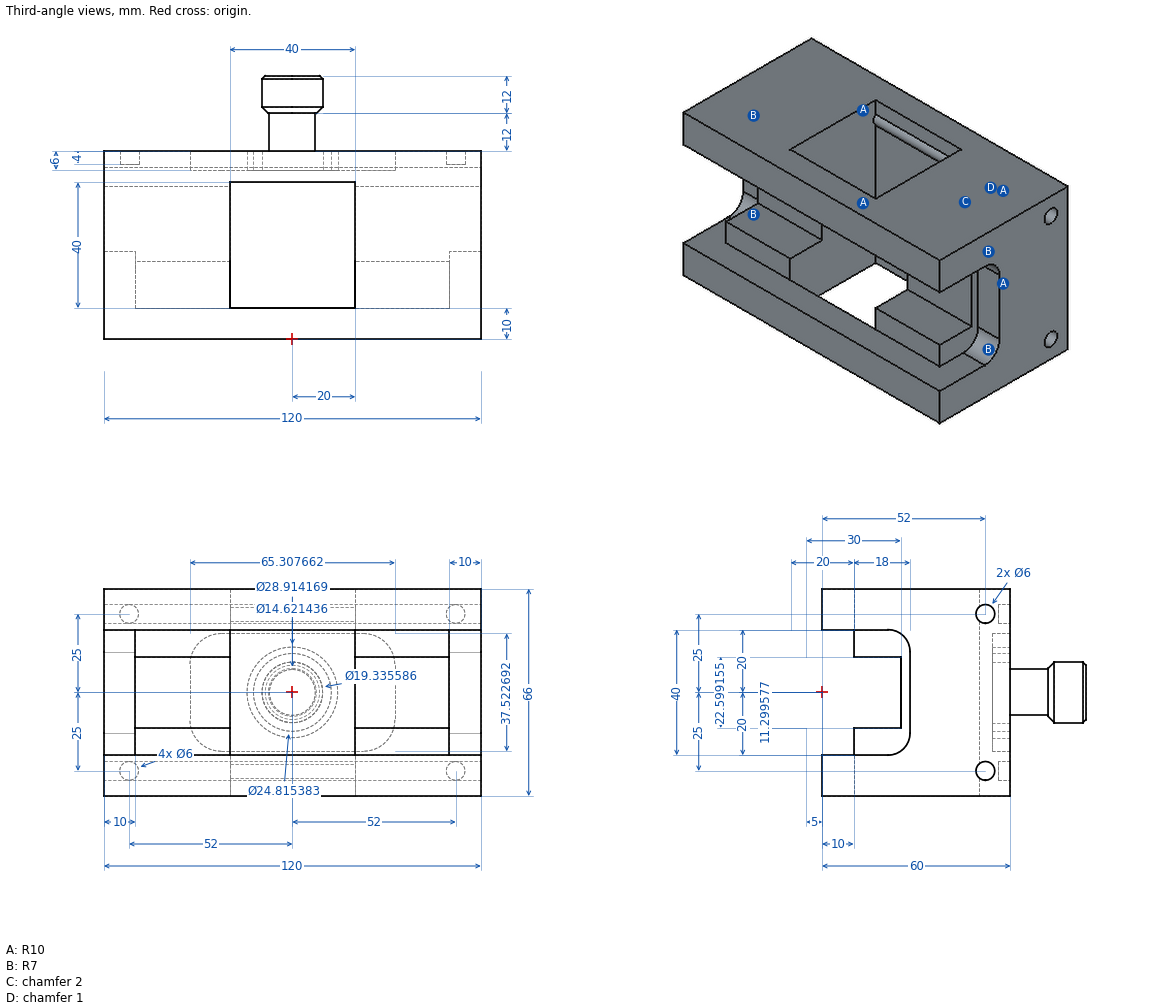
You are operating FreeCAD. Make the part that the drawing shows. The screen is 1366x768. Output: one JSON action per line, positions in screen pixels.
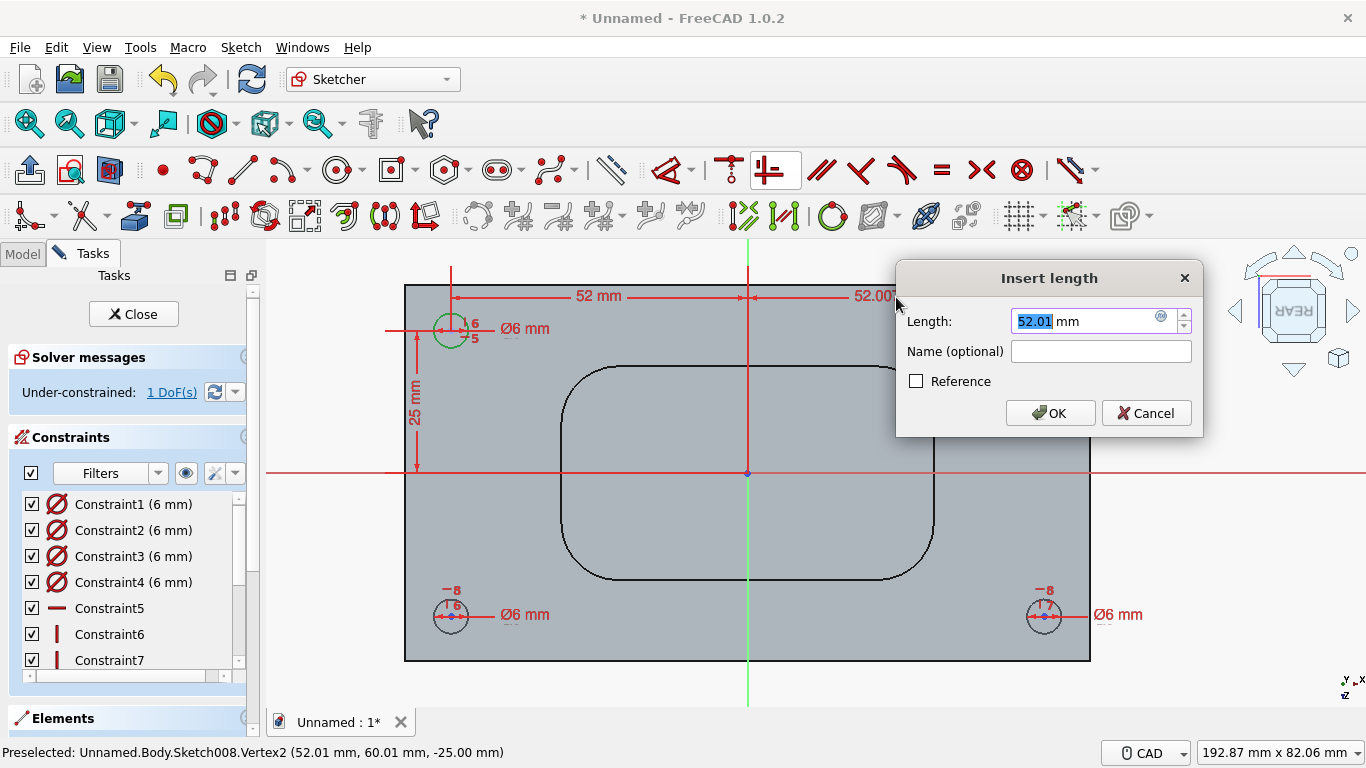
{"action": "type", "text": "52"}
{"action": "key", "text": "Return"}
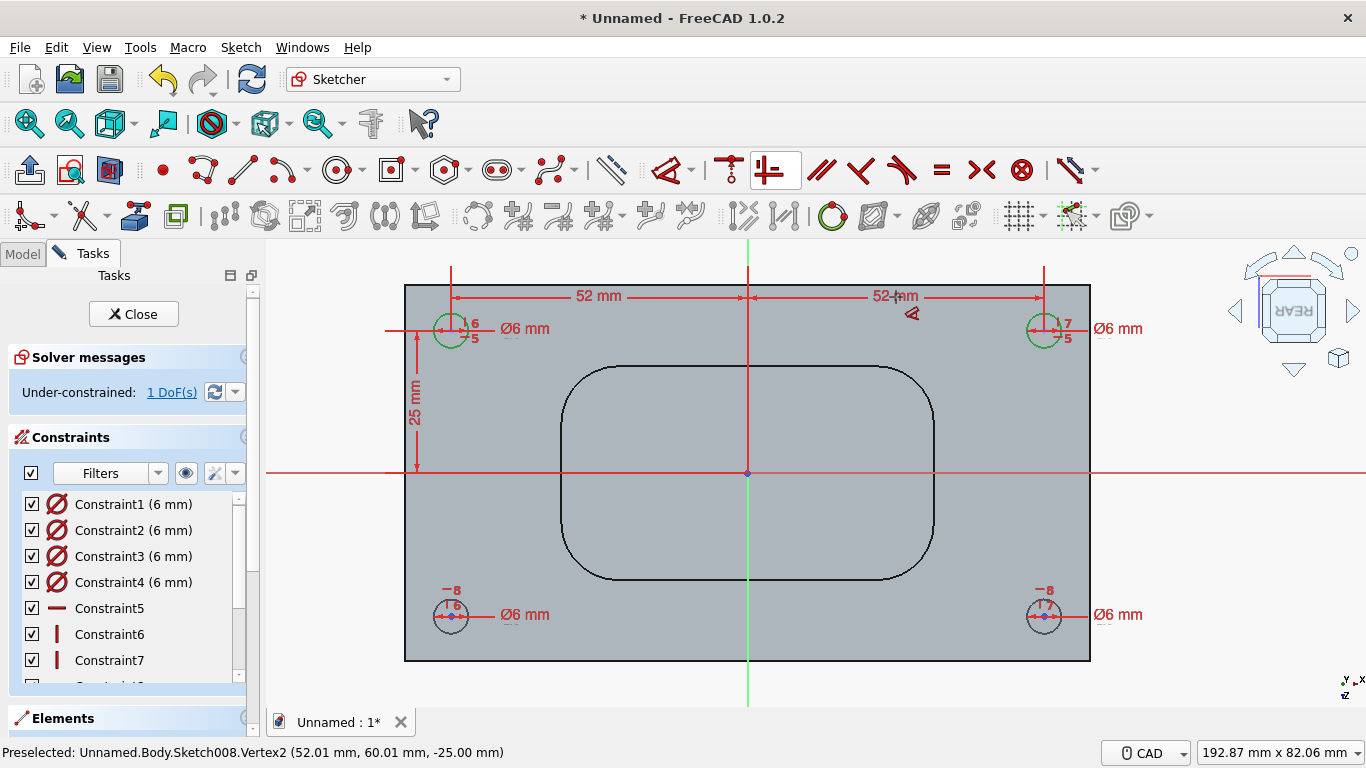
{"action": "left_click", "coordinate": [451, 617]}
{"action": "left_click", "coordinate": [417, 545]}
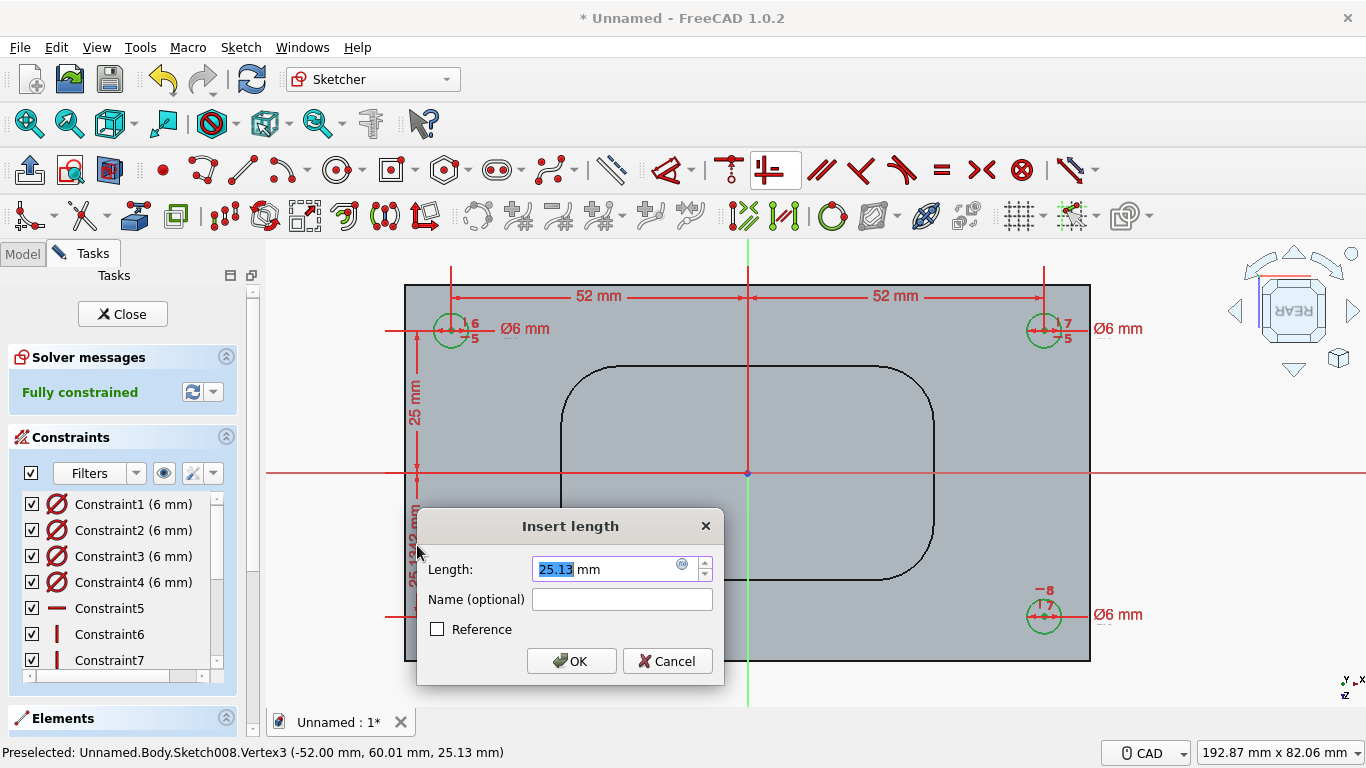
{"action": "type", "text": "25"}
{"action": "key", "text": "Return"}
{"action": "key", "text": "Escape"}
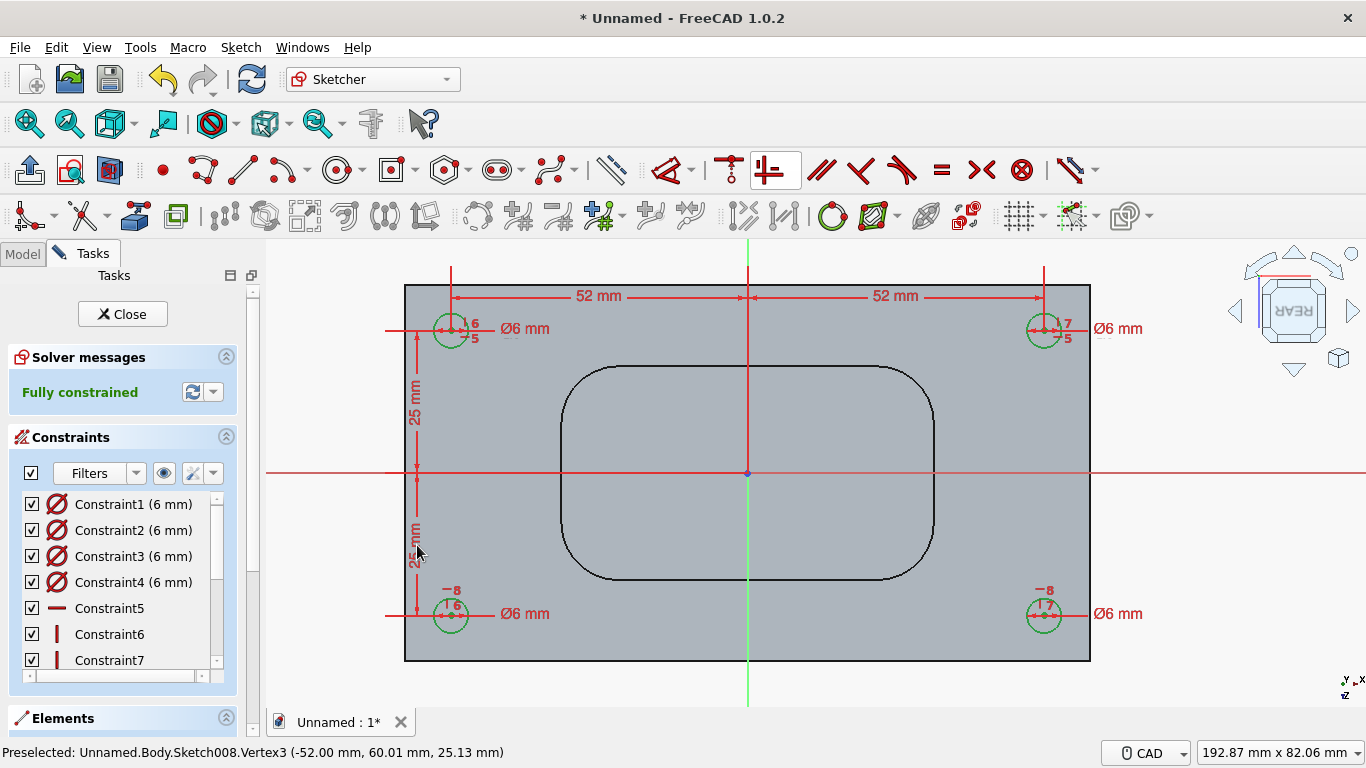
{"action": "left_click", "coordinate": [123, 314]}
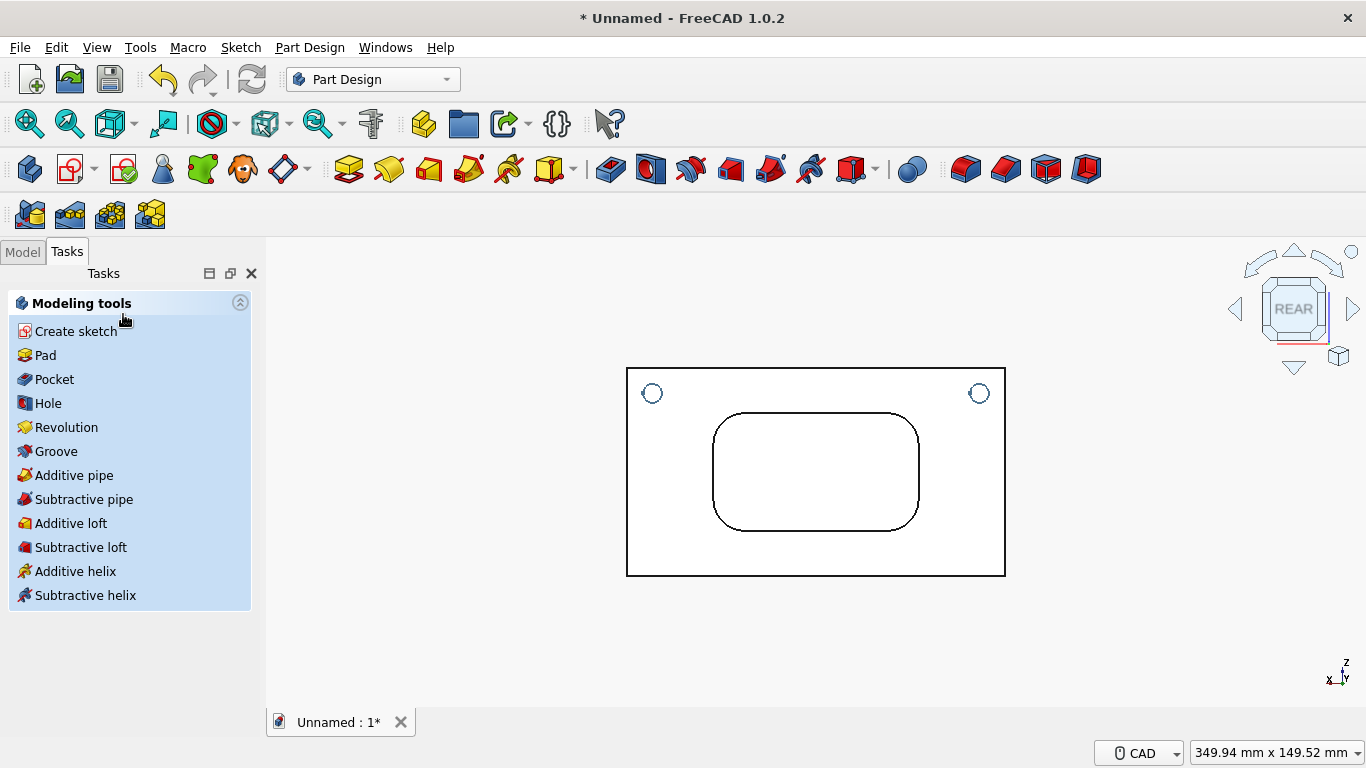
{"action": "left_click", "coordinate": [612, 170]}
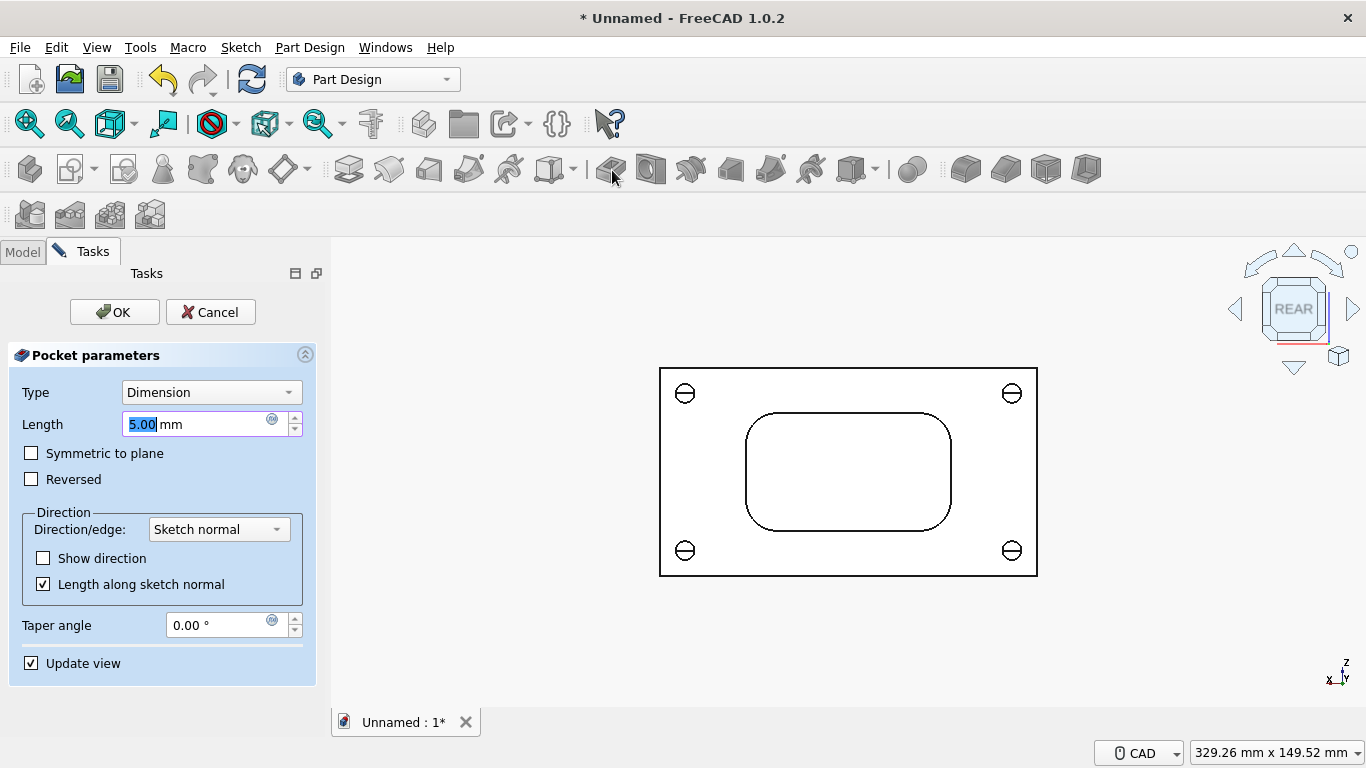
{"action": "type", "text": "4"}
{"action": "key", "text": "Tab"}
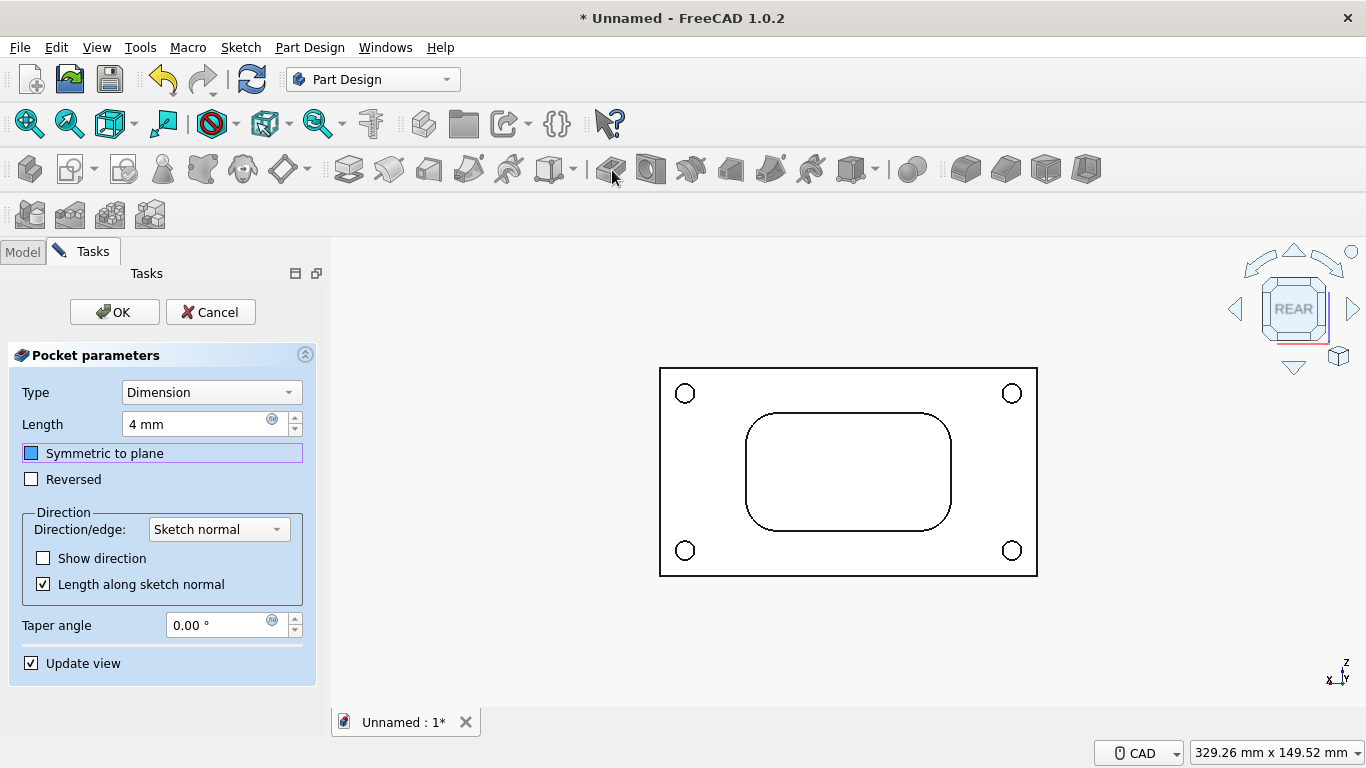
{"action": "left_click", "coordinate": [115, 312]}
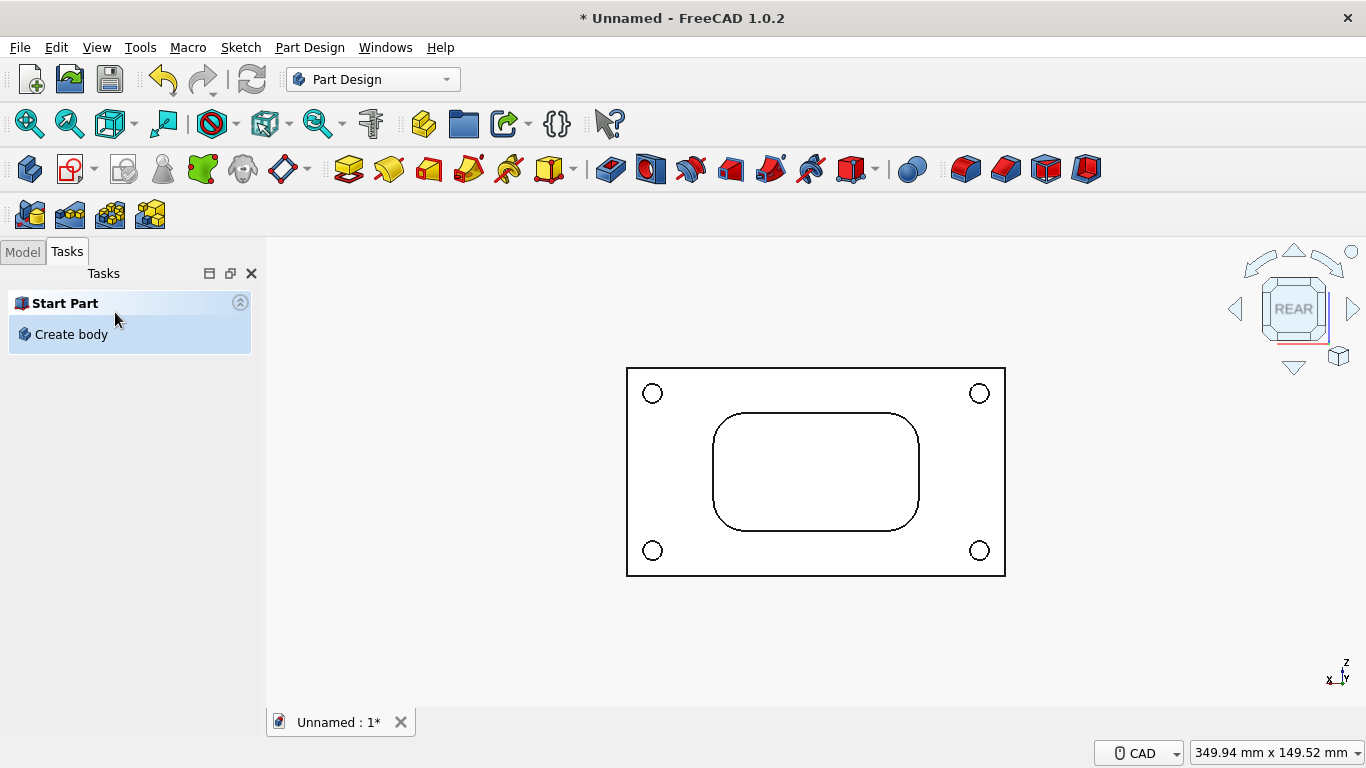
{"action": "left_click", "coordinate": [30, 124]}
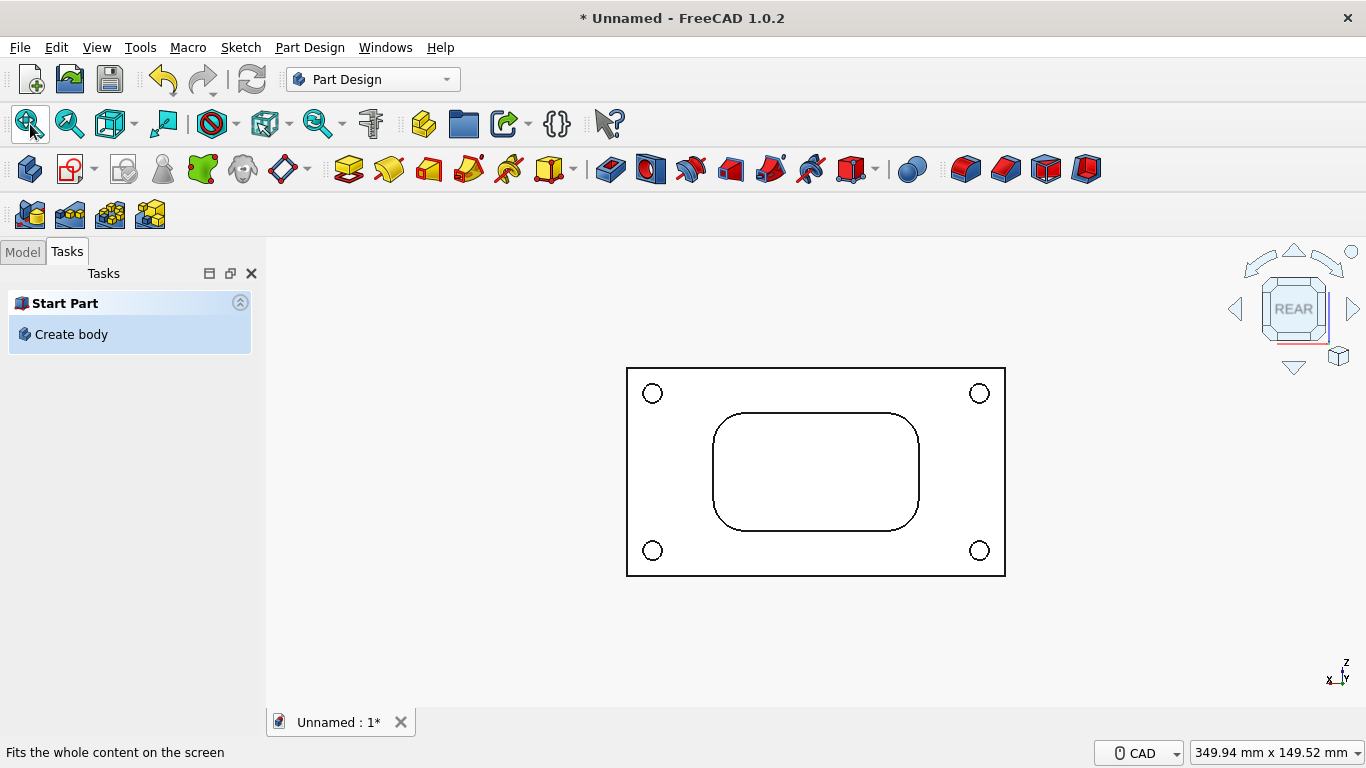
{"action": "key", "text": "0"}